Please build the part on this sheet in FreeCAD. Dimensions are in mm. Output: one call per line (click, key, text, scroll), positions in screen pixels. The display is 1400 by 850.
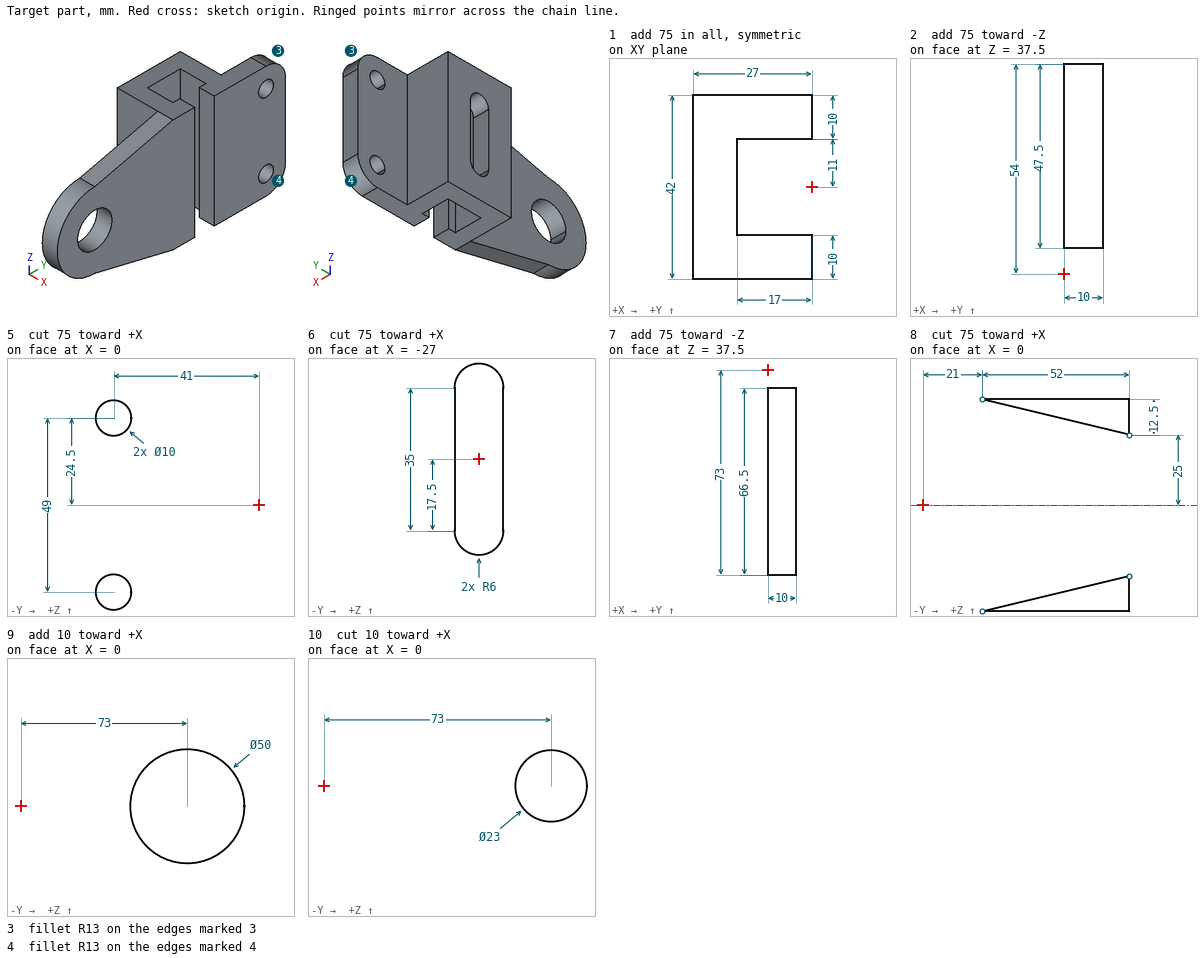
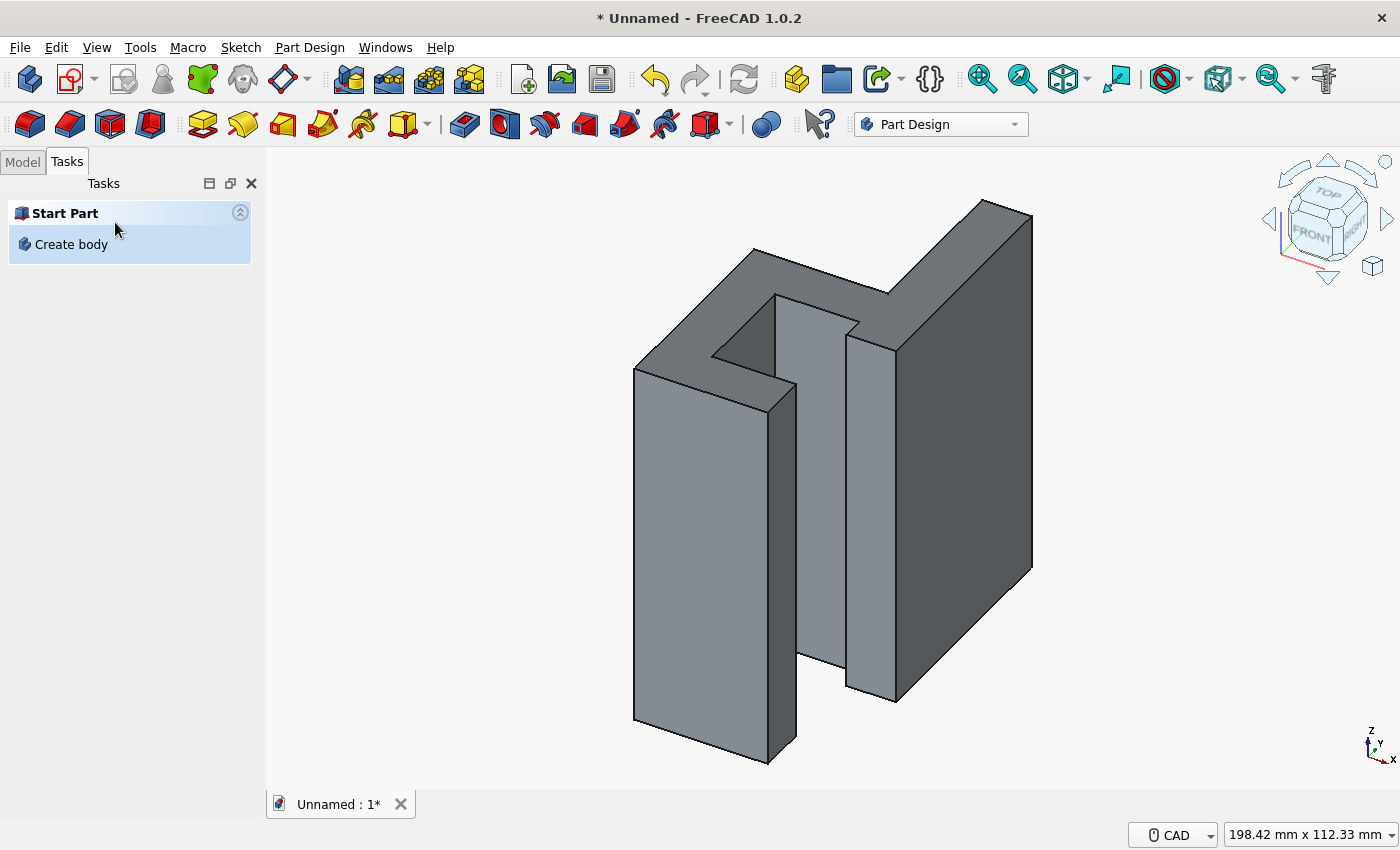
key(0)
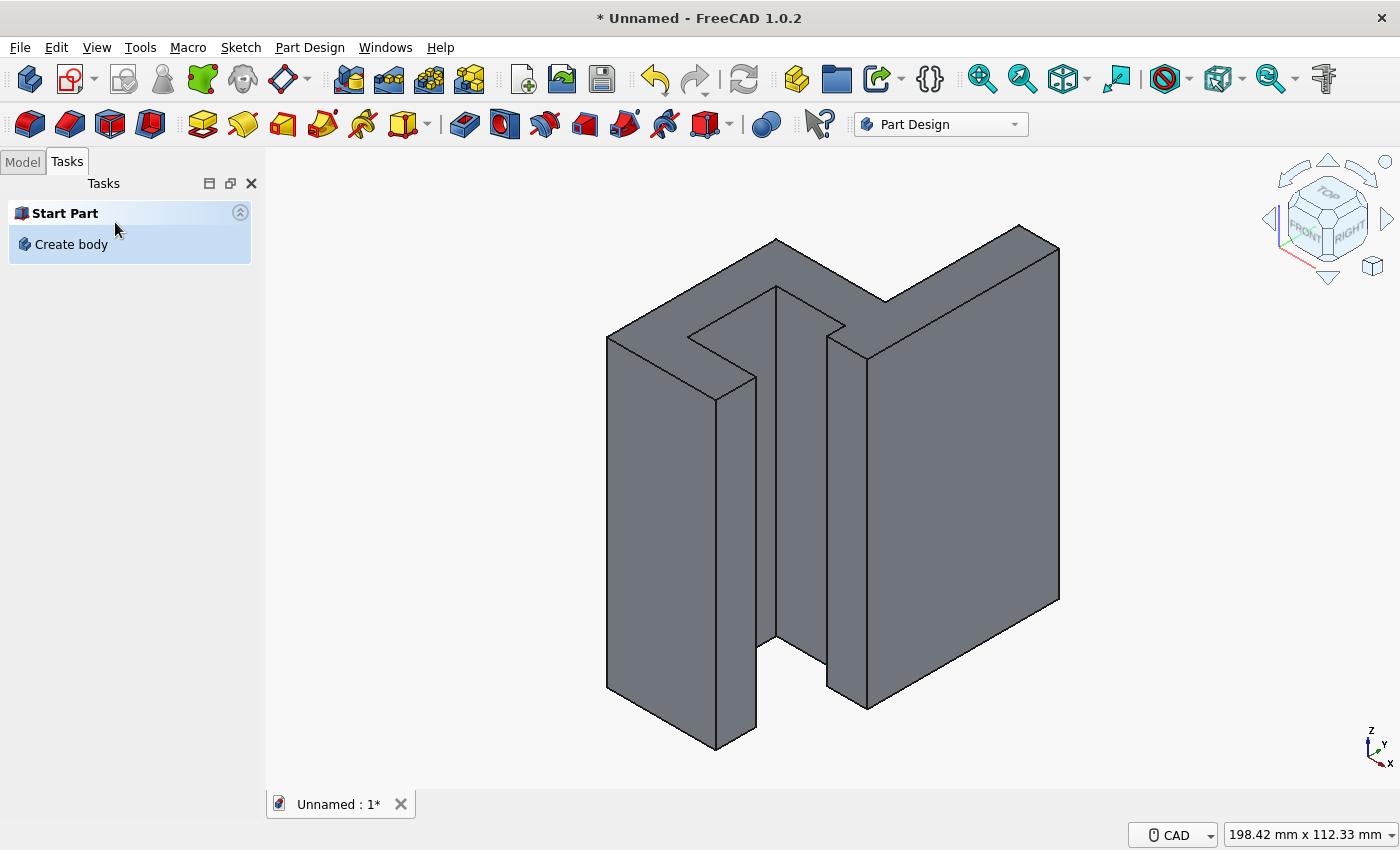
key(2)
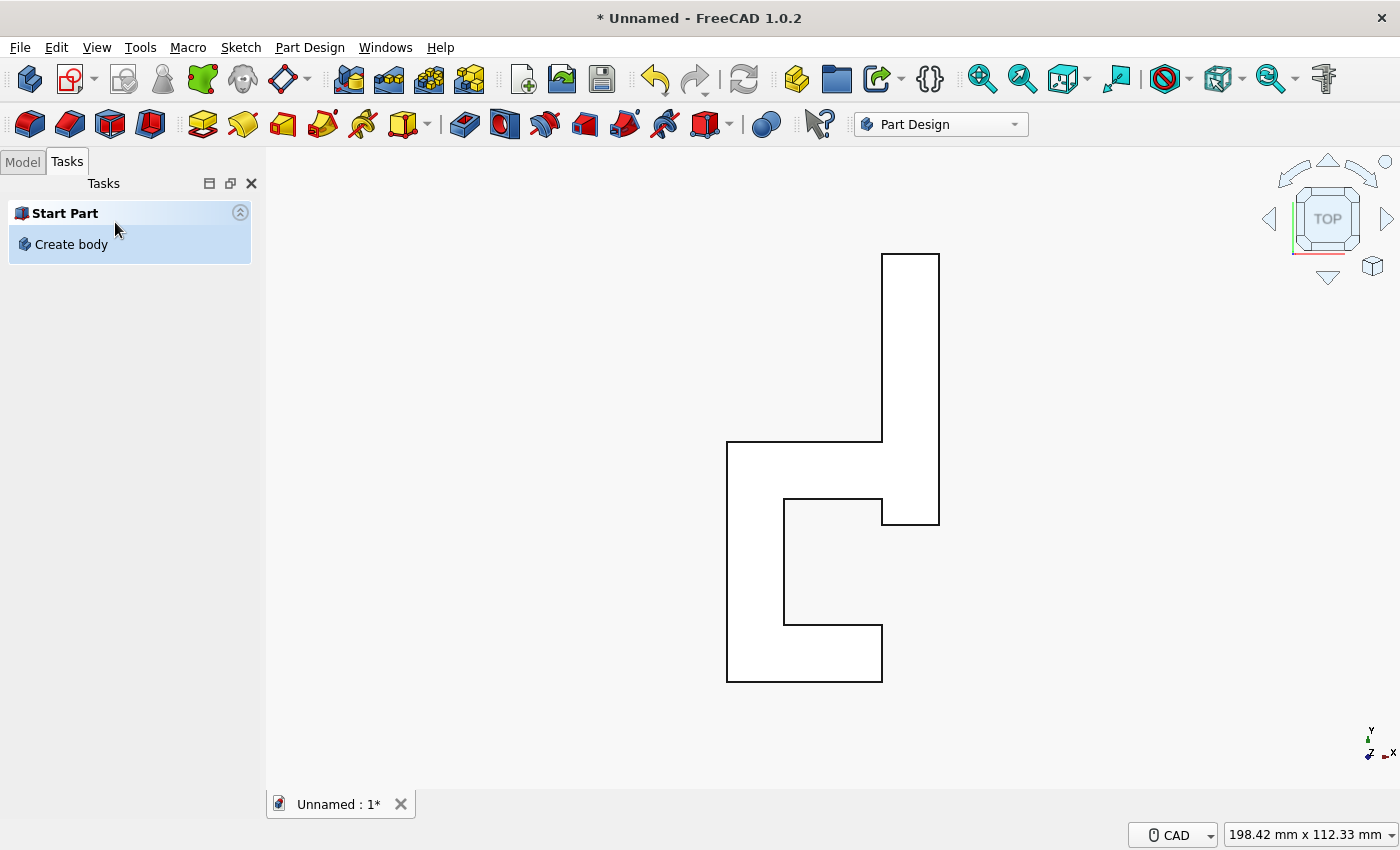
click(910, 253)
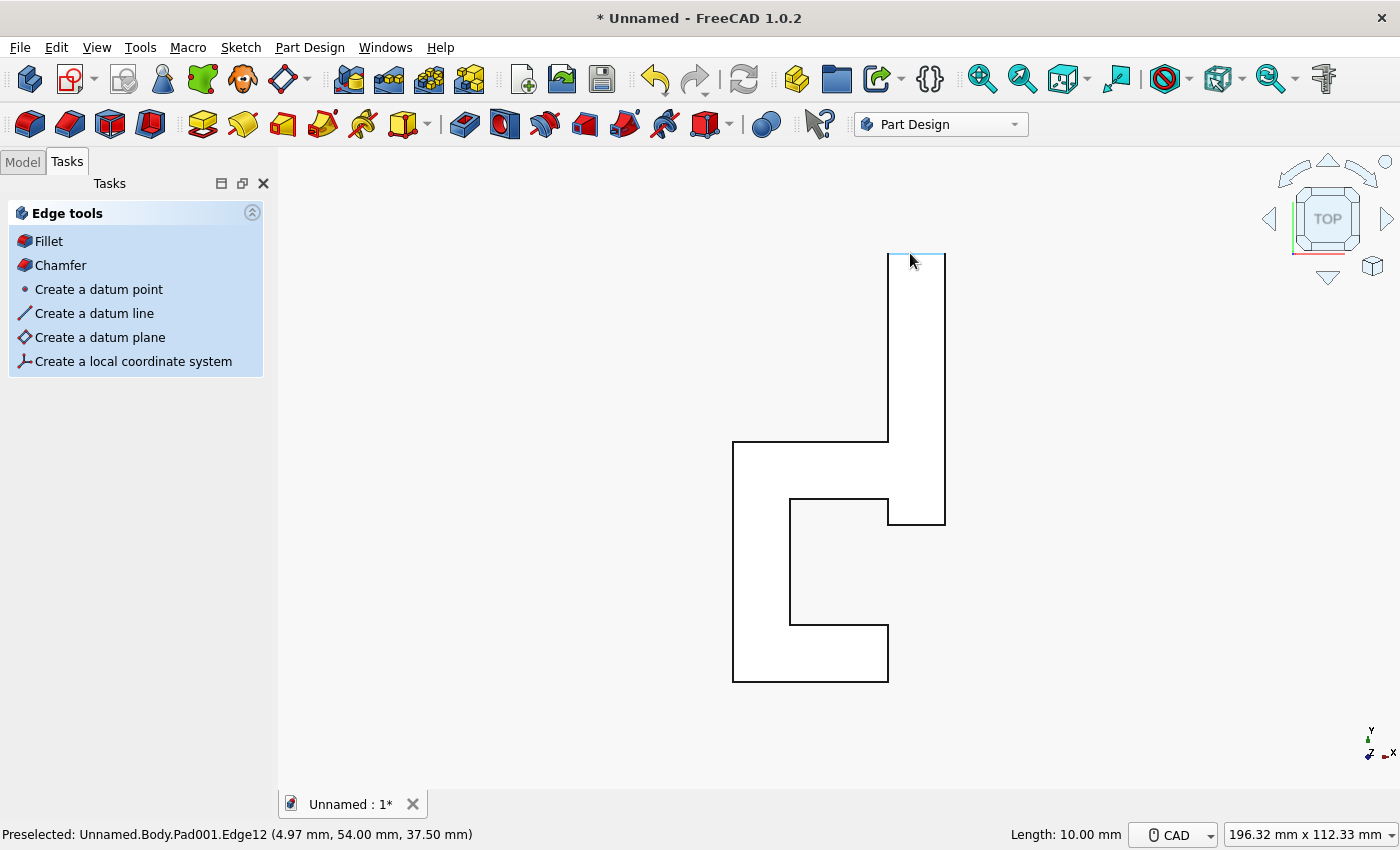
click(30, 124)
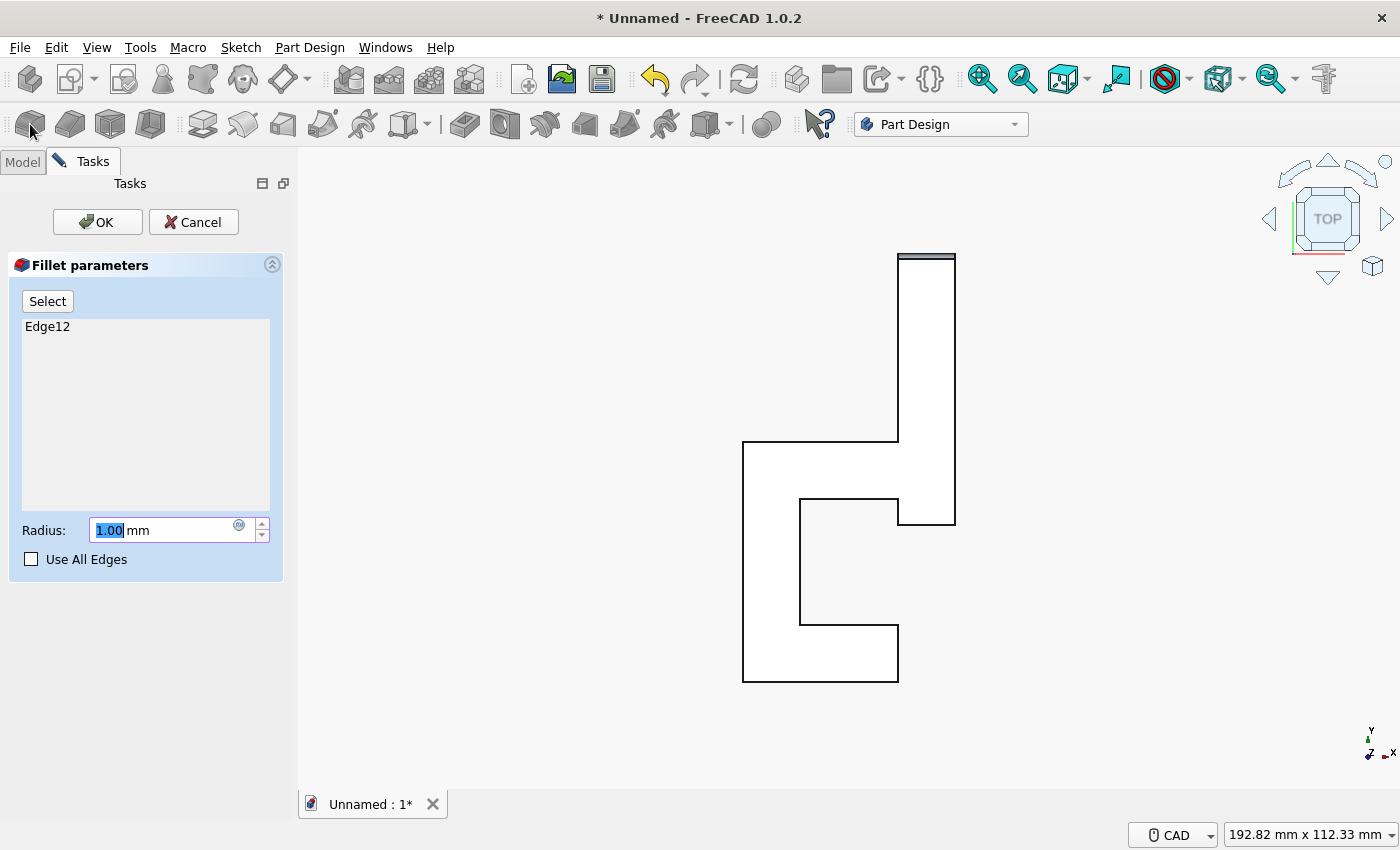
text(13)
key(Tab)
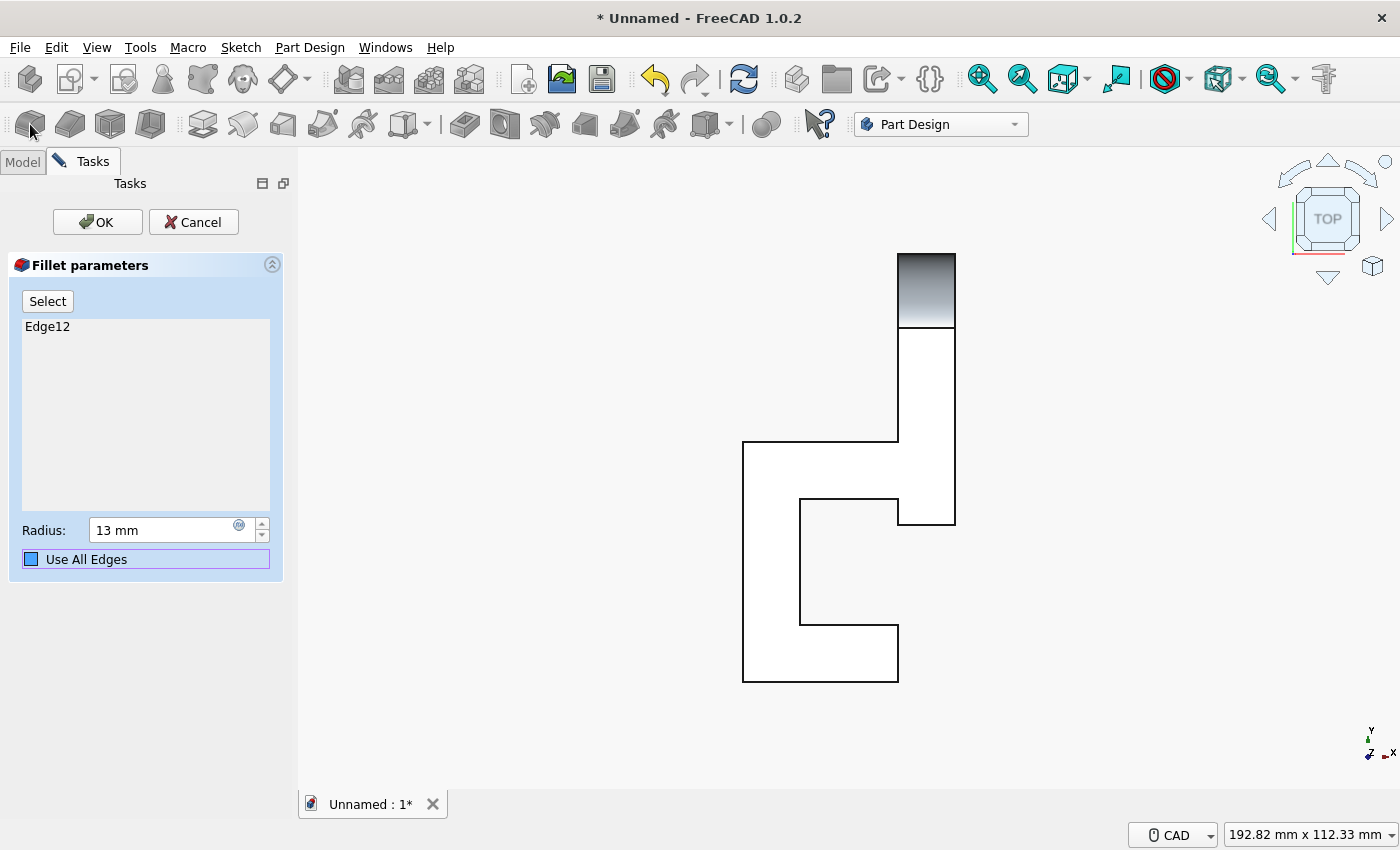
click(98, 222)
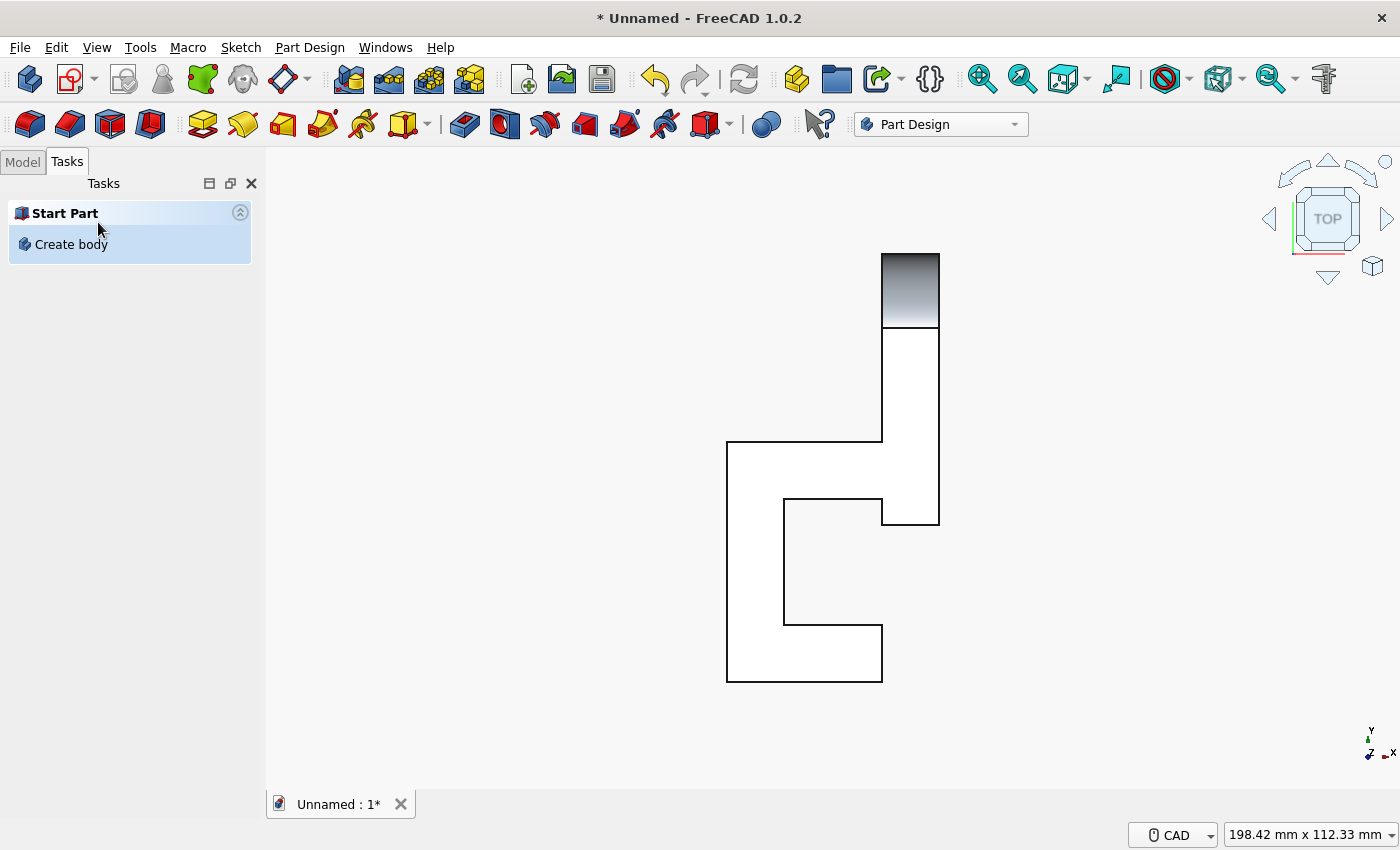
key(0)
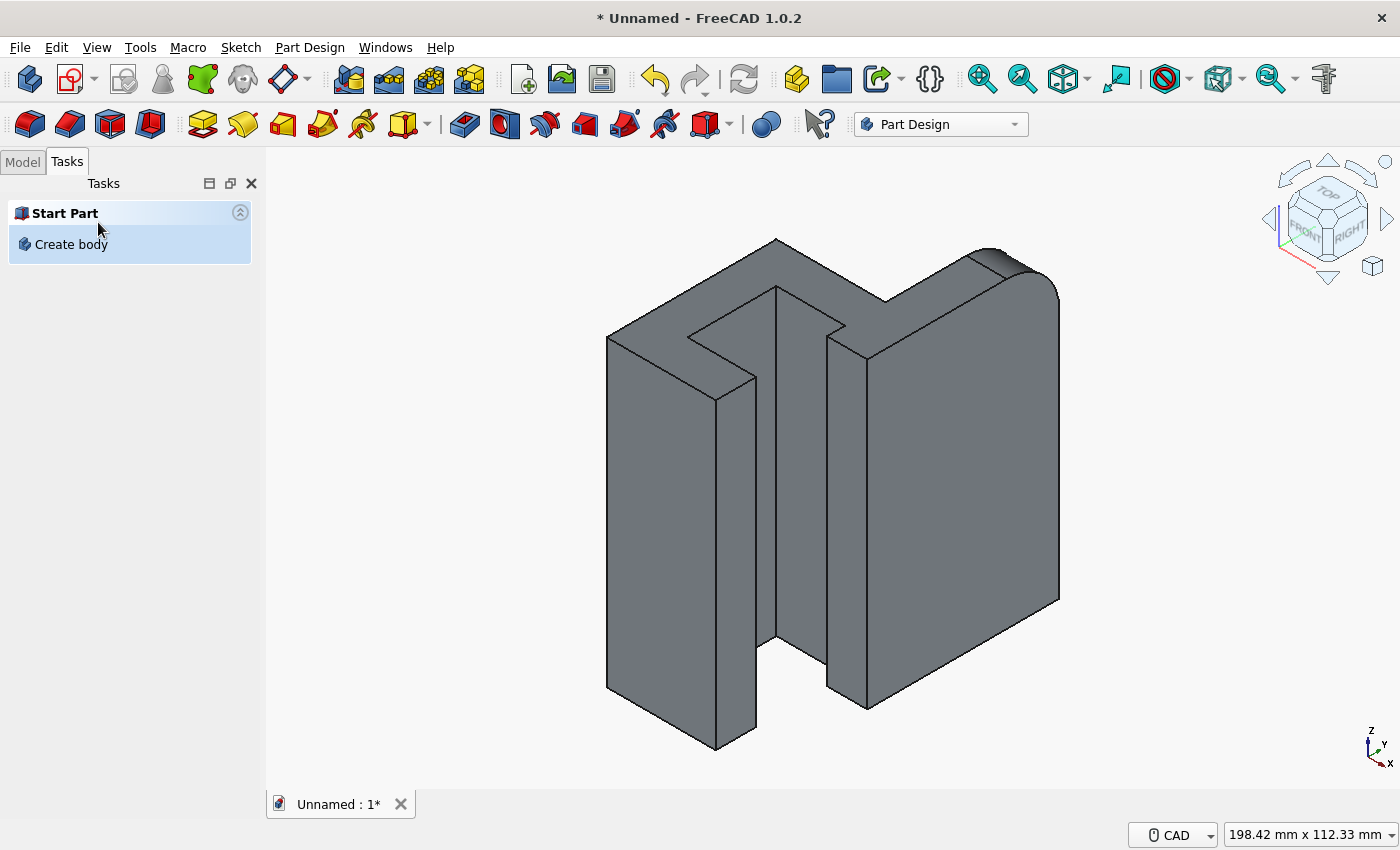
key(2)